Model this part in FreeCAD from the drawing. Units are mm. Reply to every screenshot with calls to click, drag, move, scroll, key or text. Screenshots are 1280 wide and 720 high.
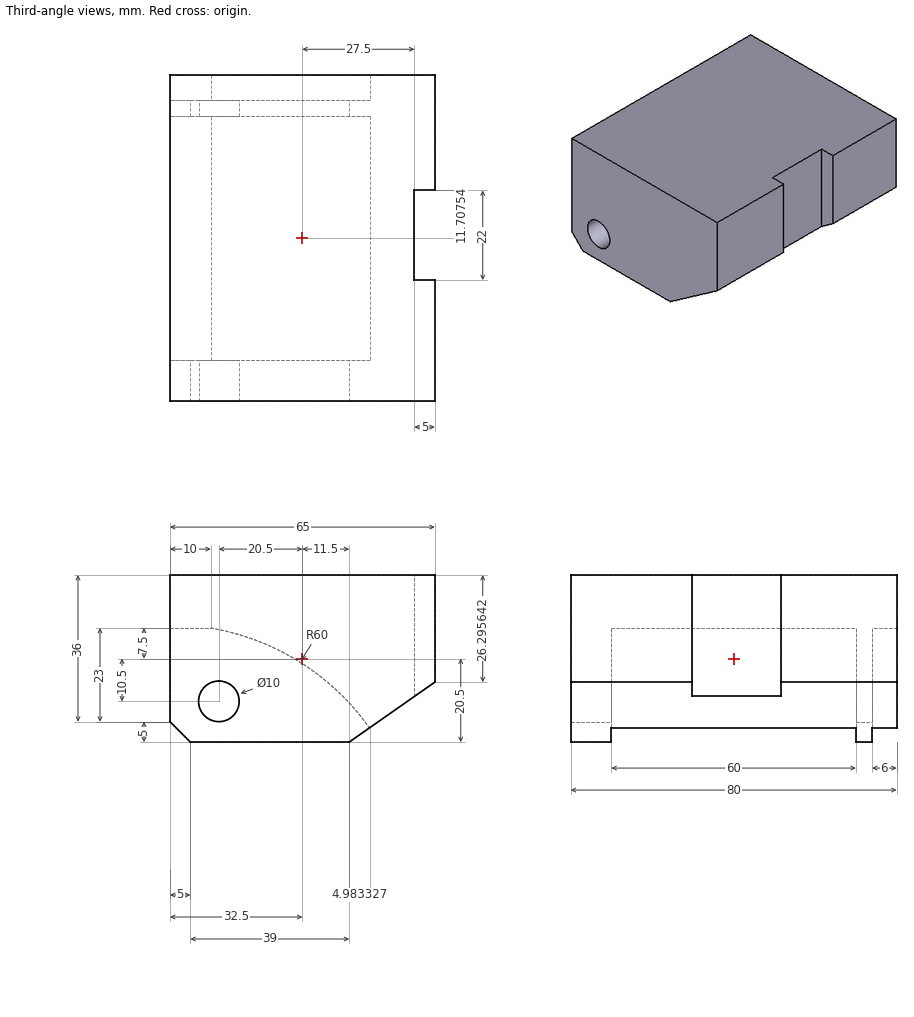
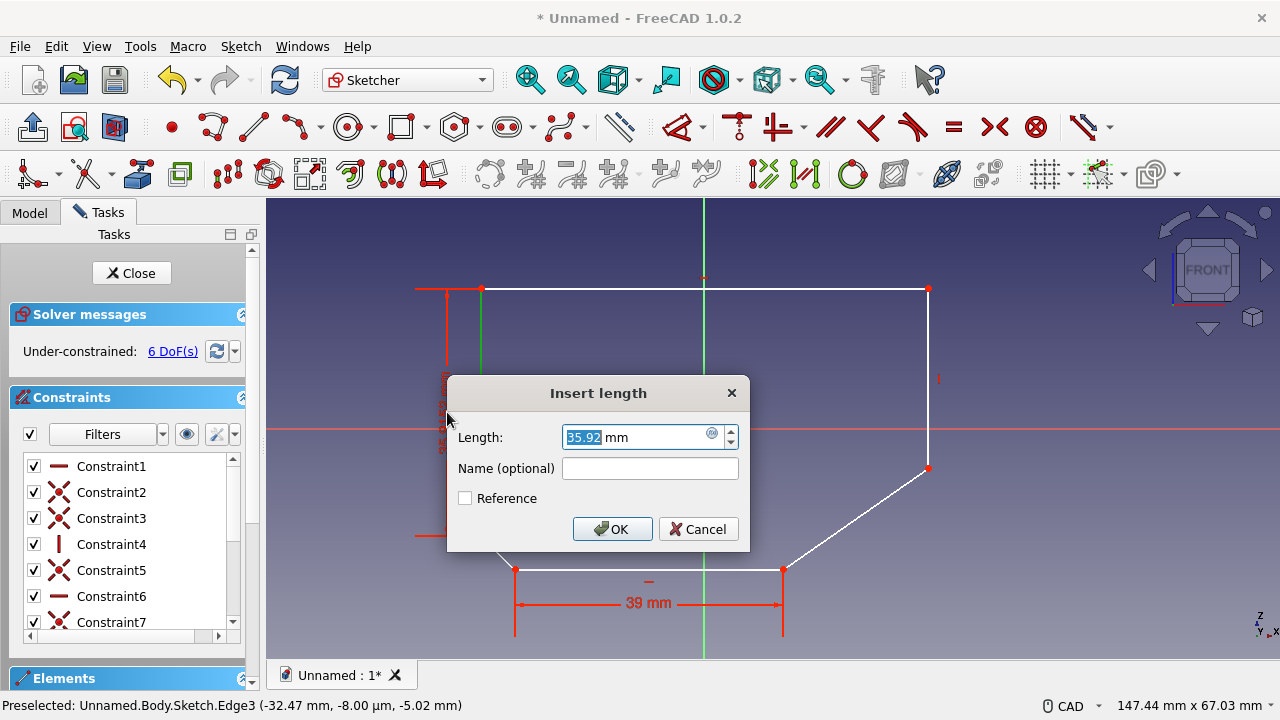
text(36)
key(Return)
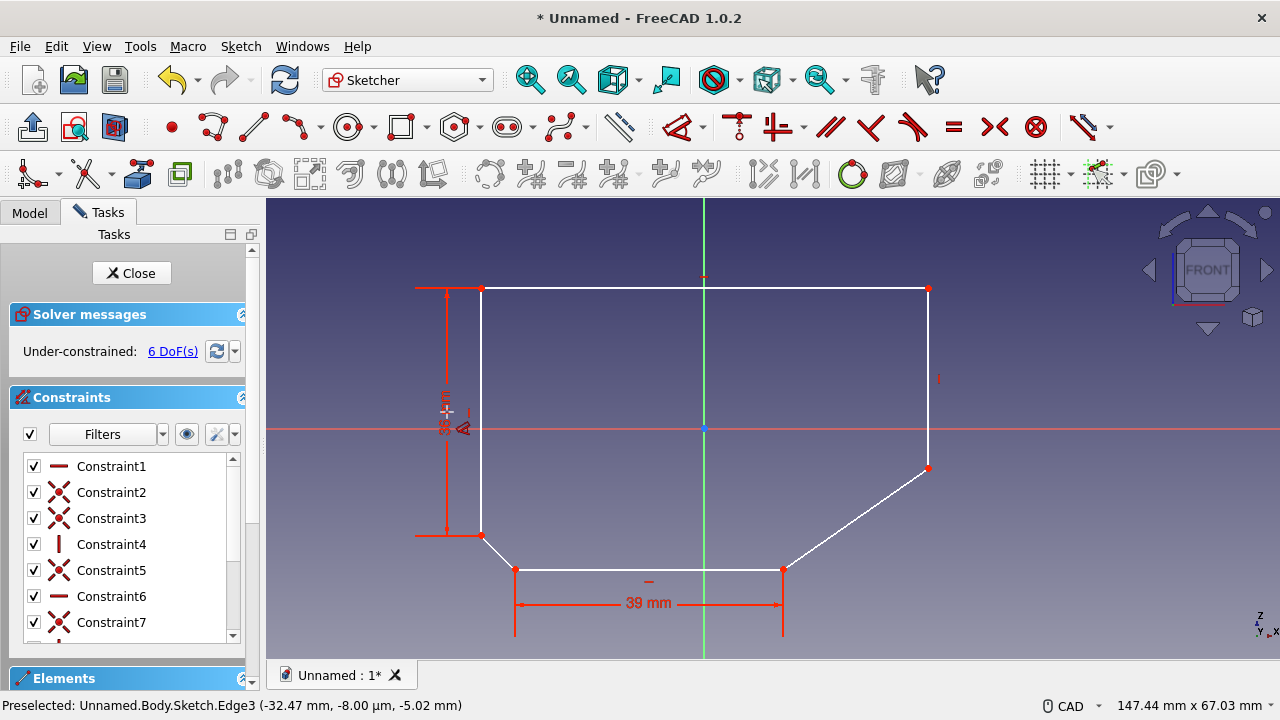
click(615, 288)
click(602, 254)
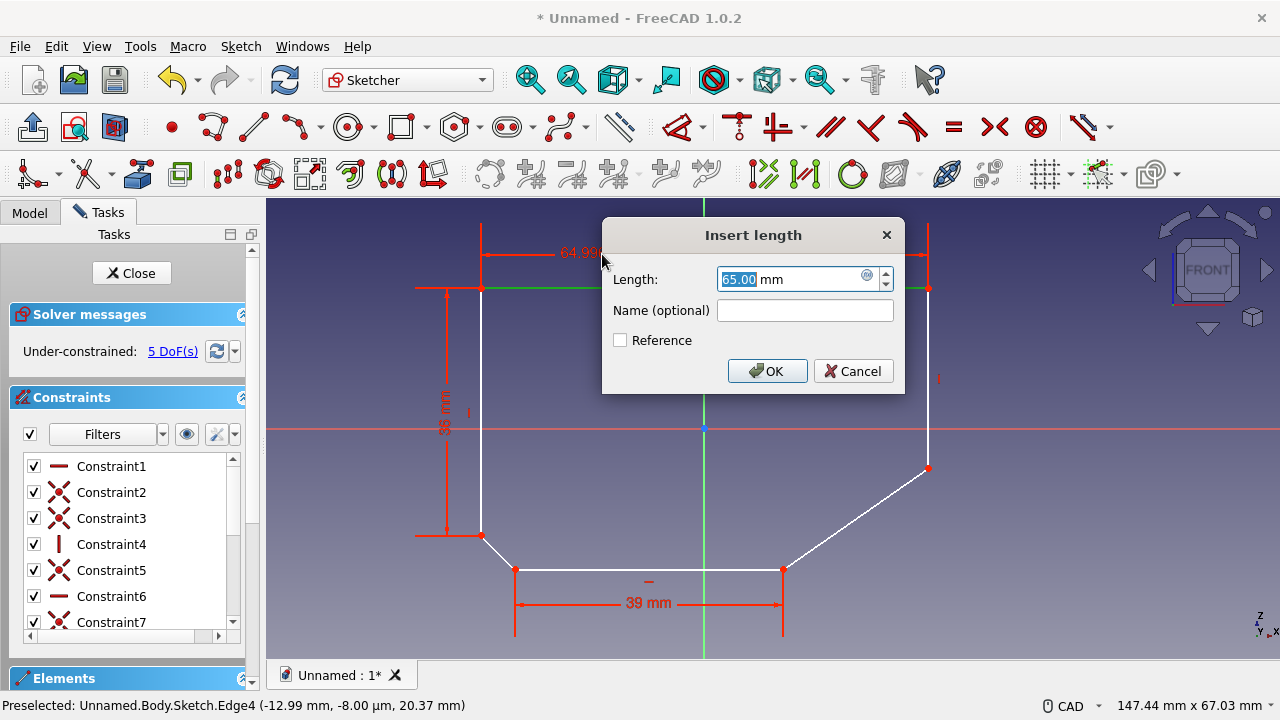
text(65)
key(Return)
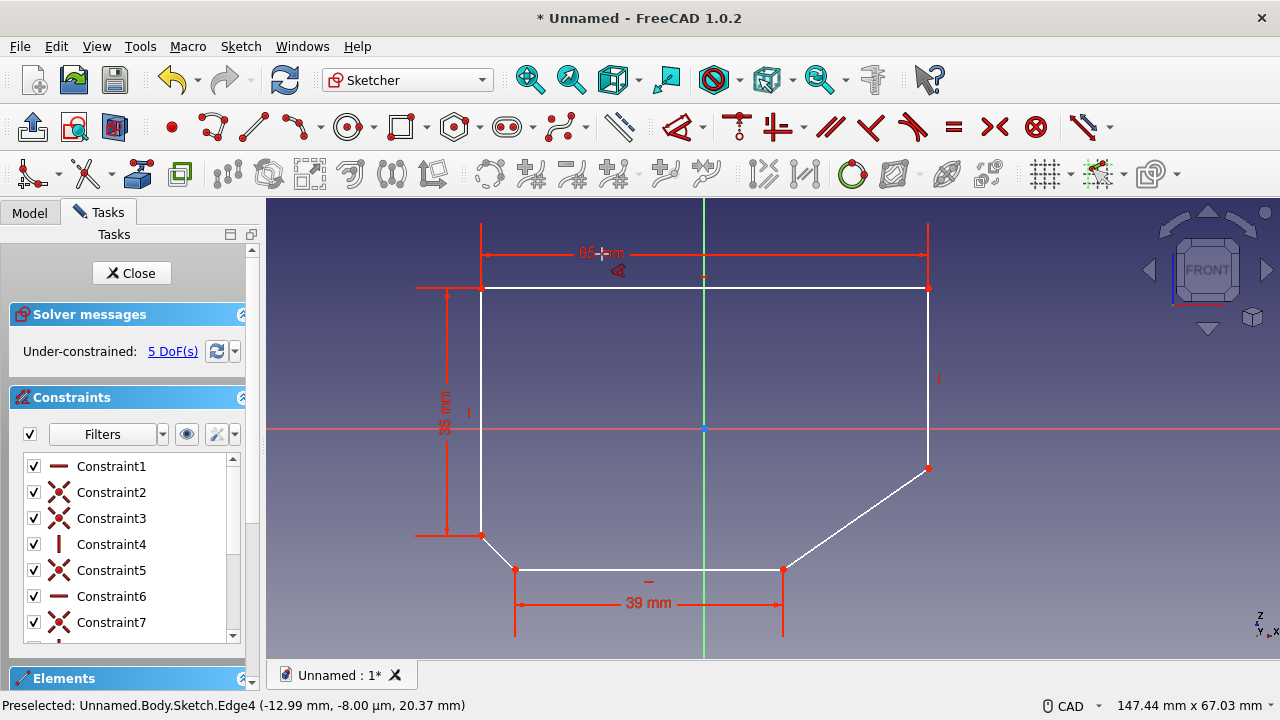
click(505, 560)
click(498, 604)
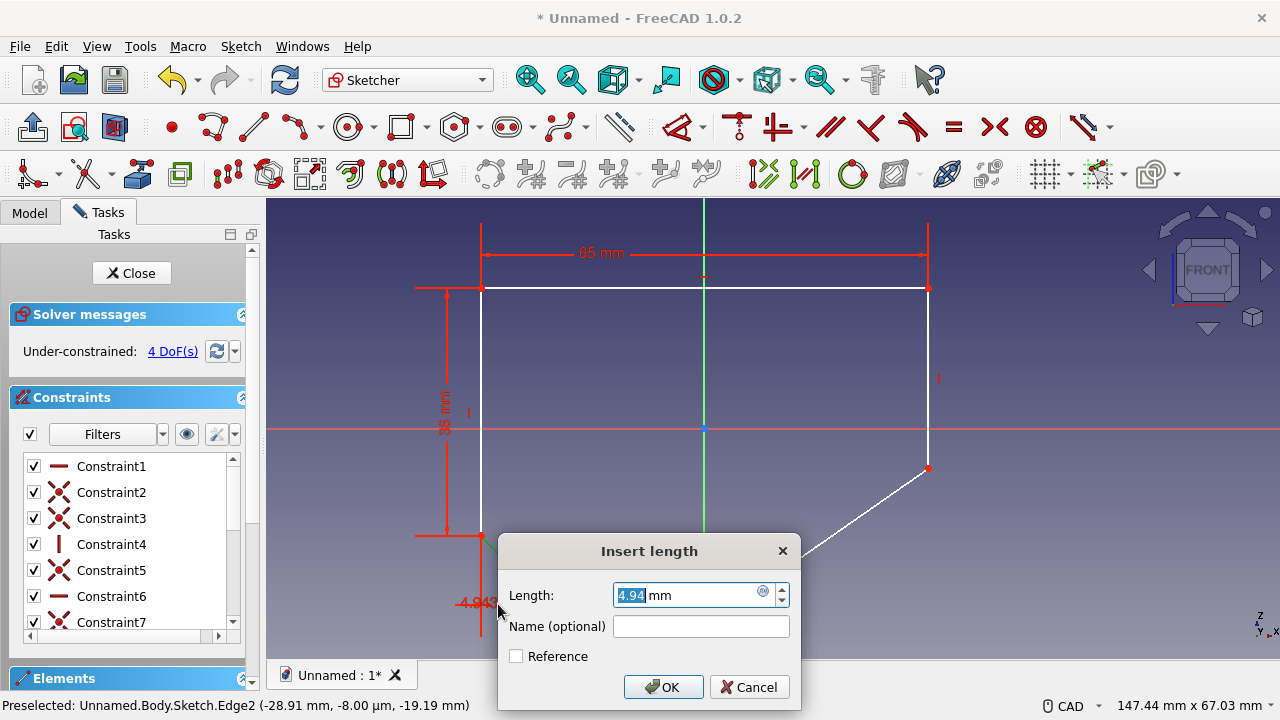
text(5)
key(Return)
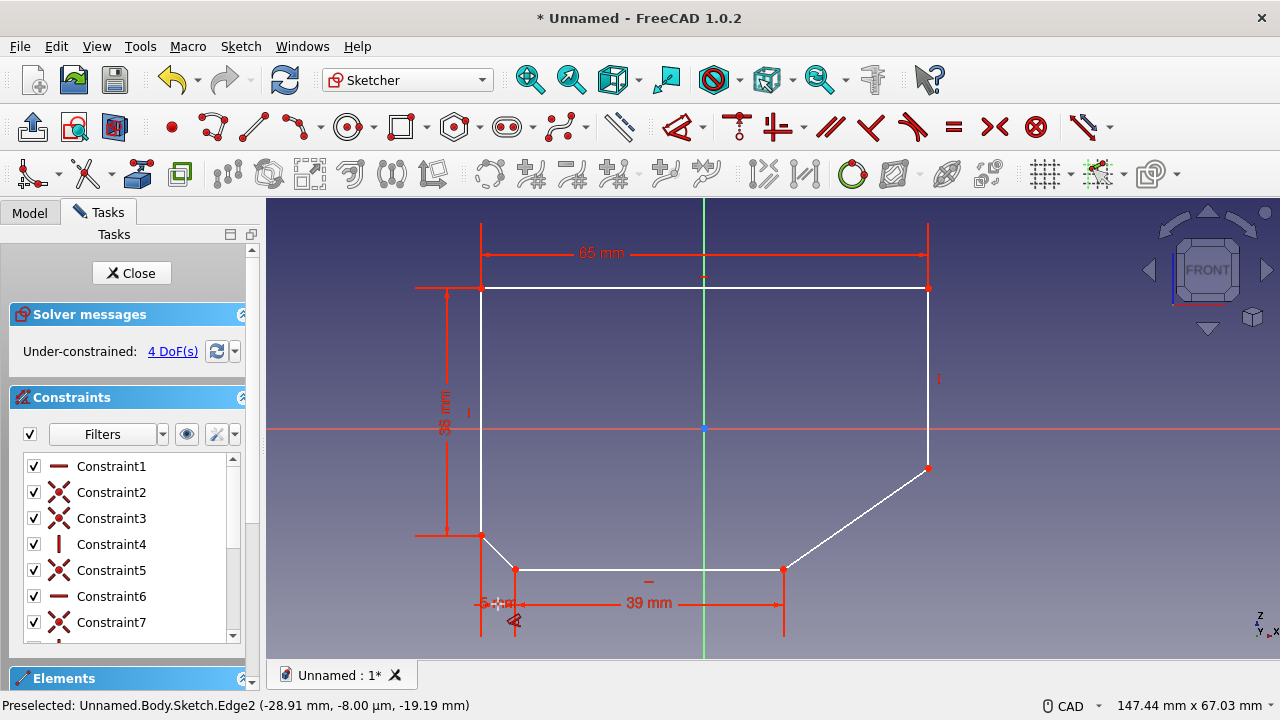
click(505, 560)
click(447, 553)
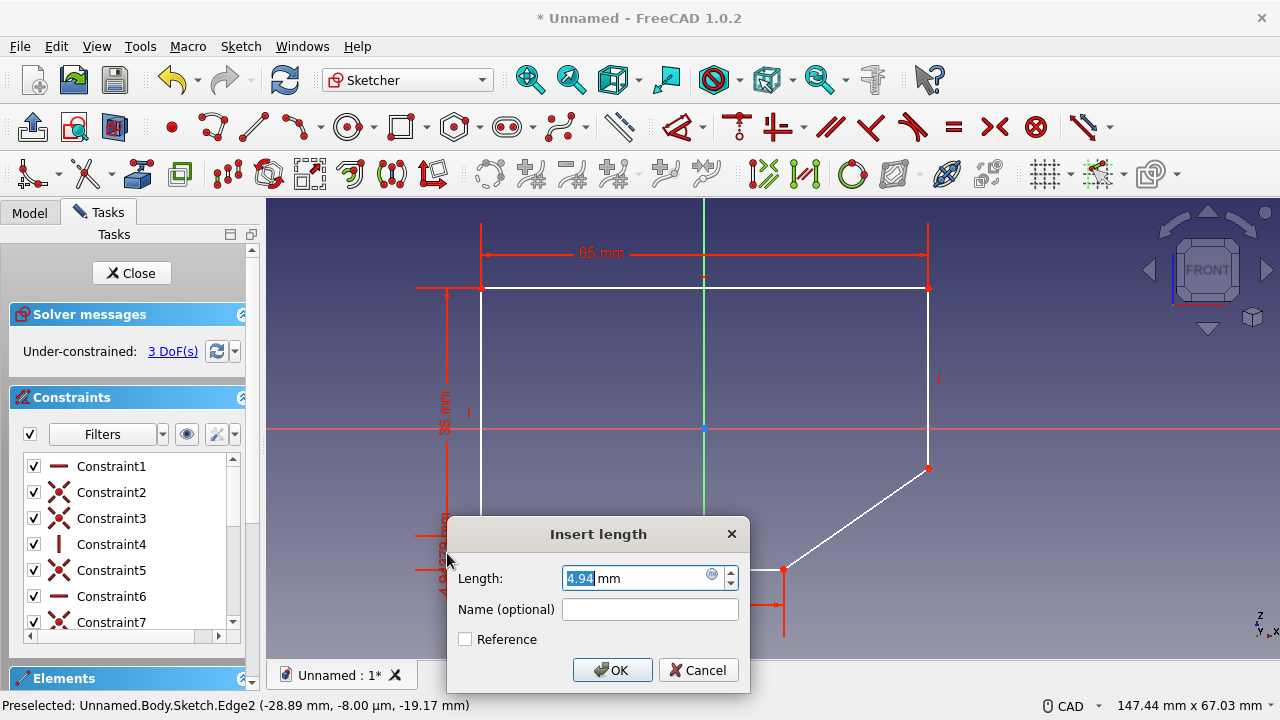
text(5)
key(Return)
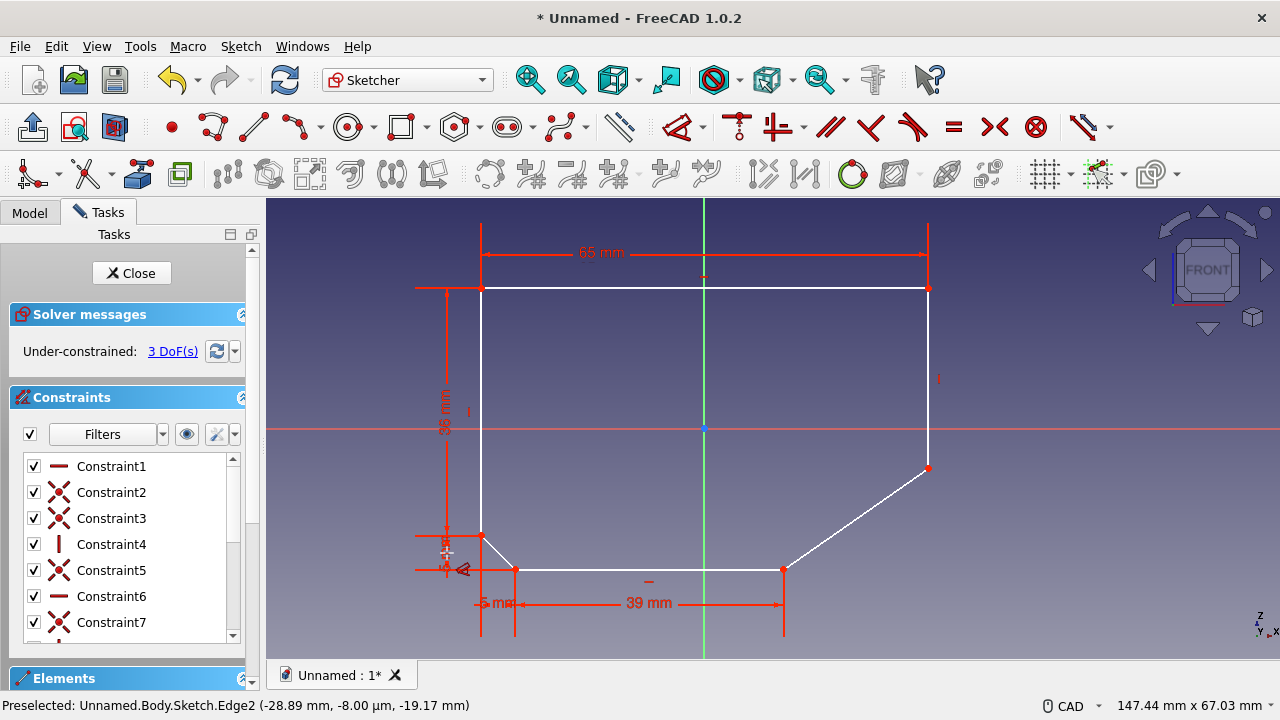
click(784, 570)
click(744, 604)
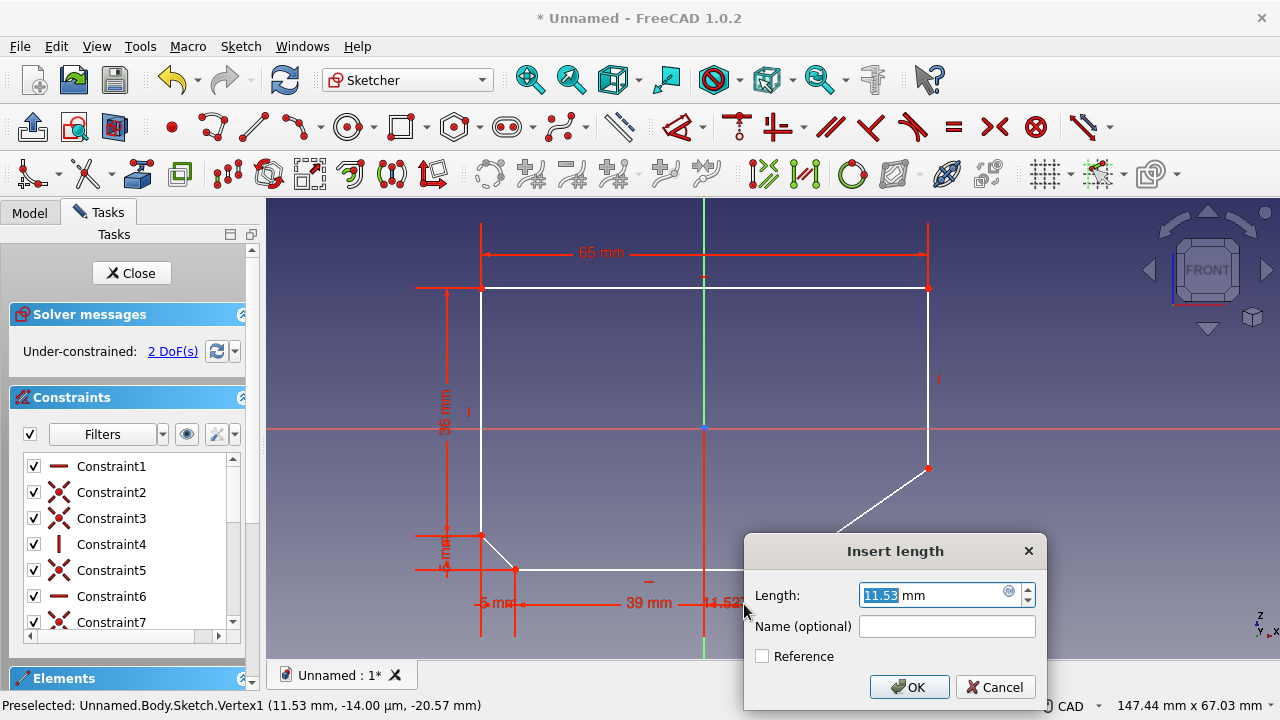
text(11.5)
key(Return)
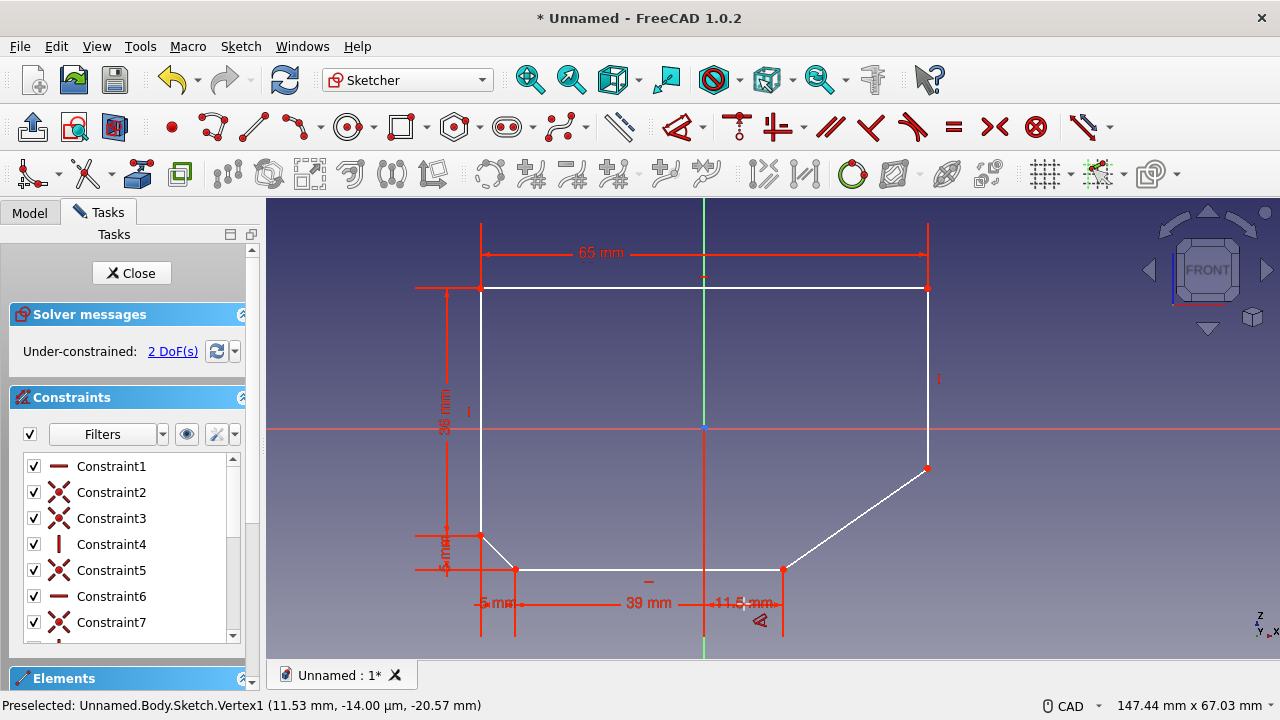
click(783, 570)
click(817, 499)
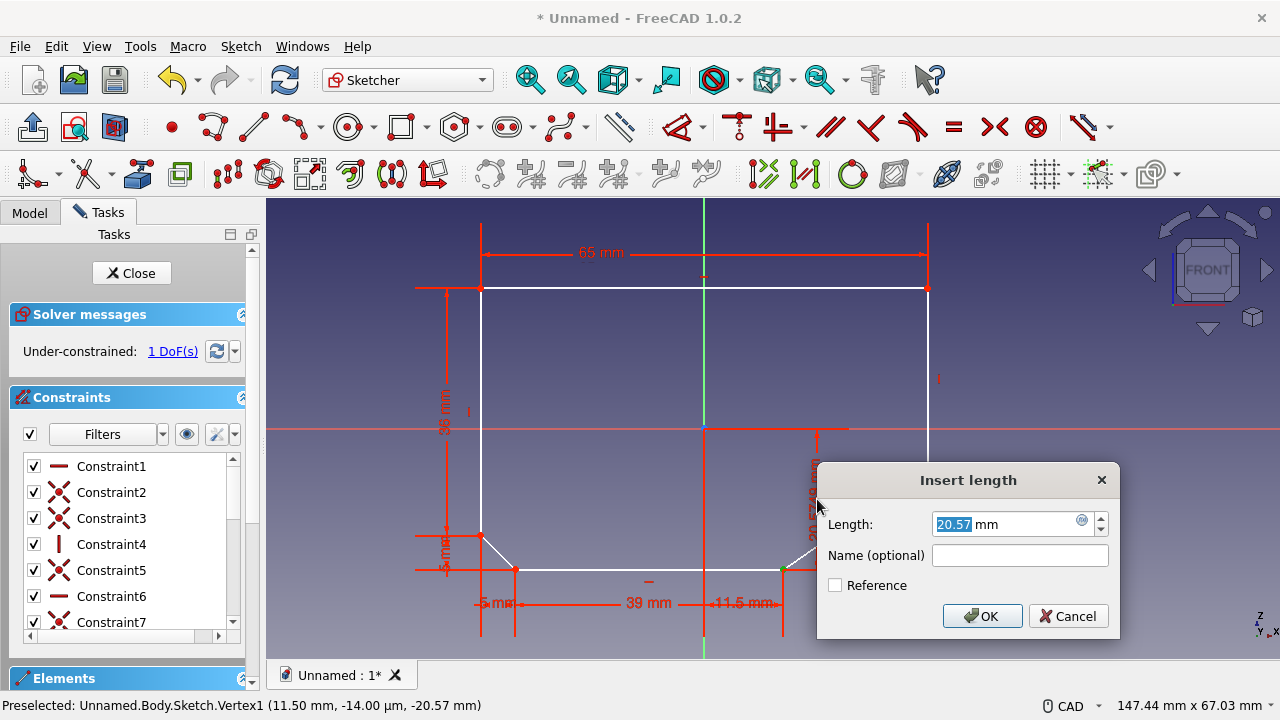
text(20.5)
key(Return)